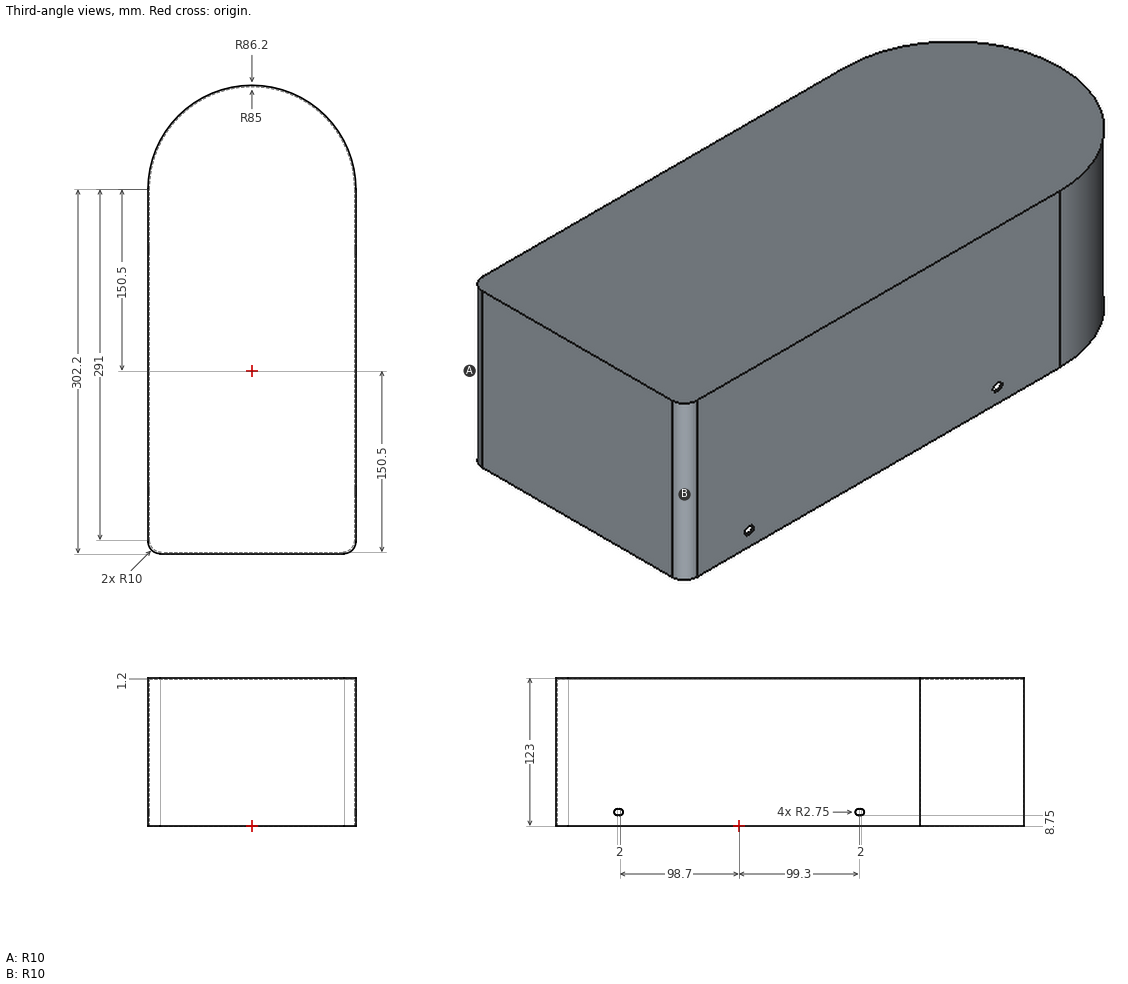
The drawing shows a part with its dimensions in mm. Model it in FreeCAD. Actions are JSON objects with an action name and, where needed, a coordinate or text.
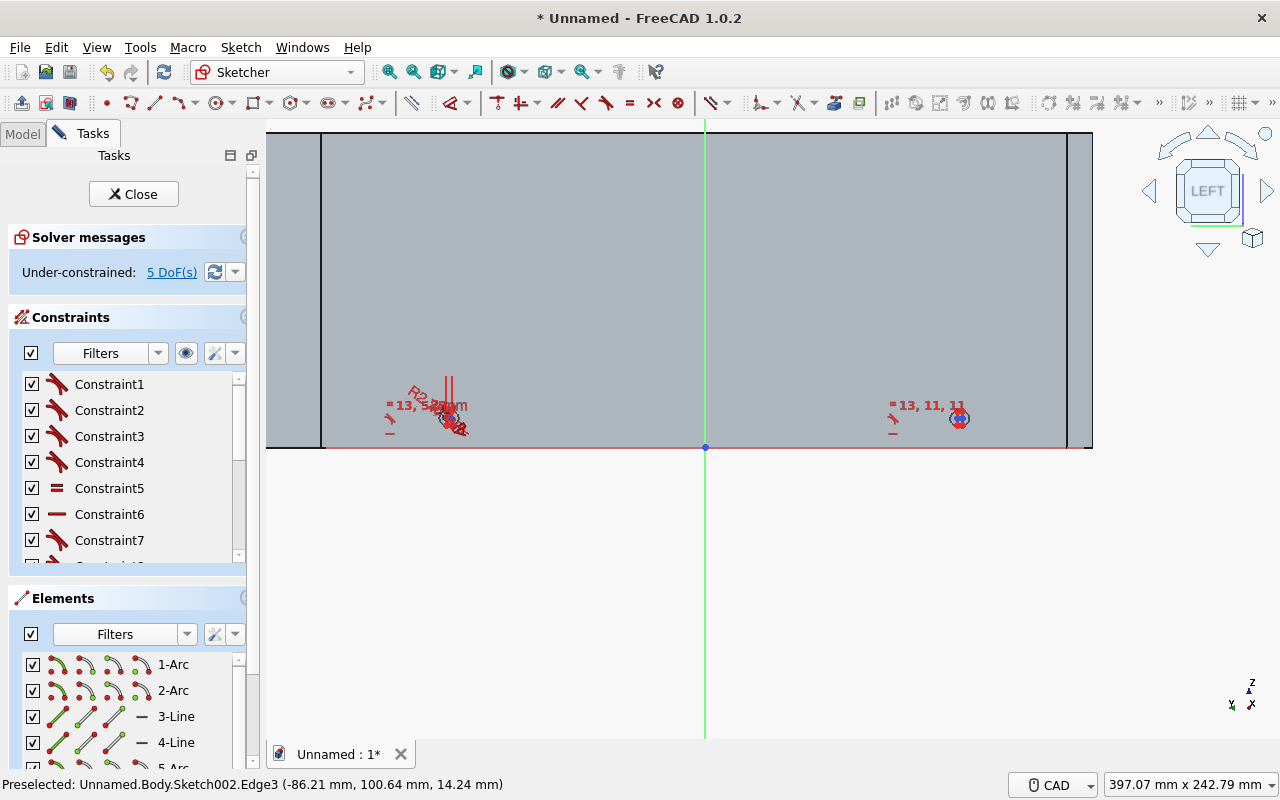
{"action": "scroll", "coordinate": [959, 412], "scroll_direction": "up", "scroll_amount": 11}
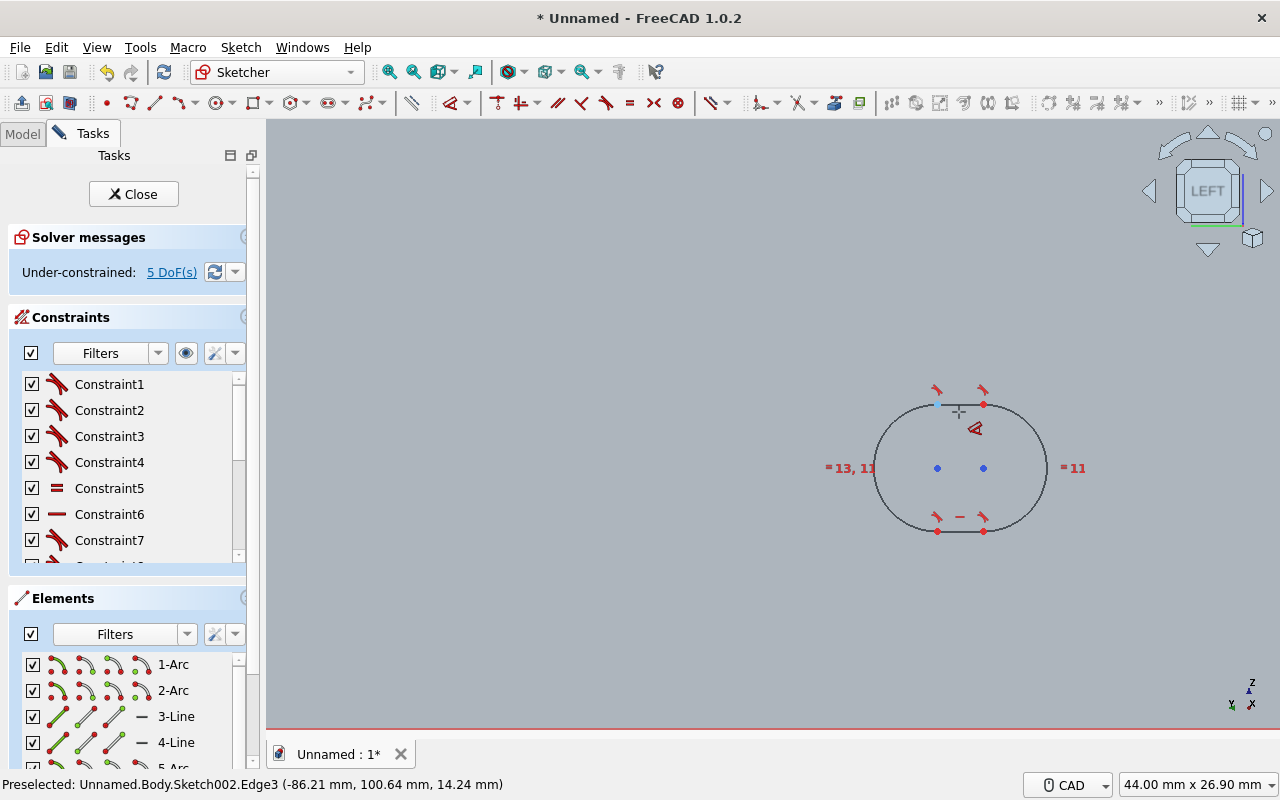
{"action": "left_click", "coordinate": [951, 405]}
{"action": "left_click", "coordinate": [960, 371]}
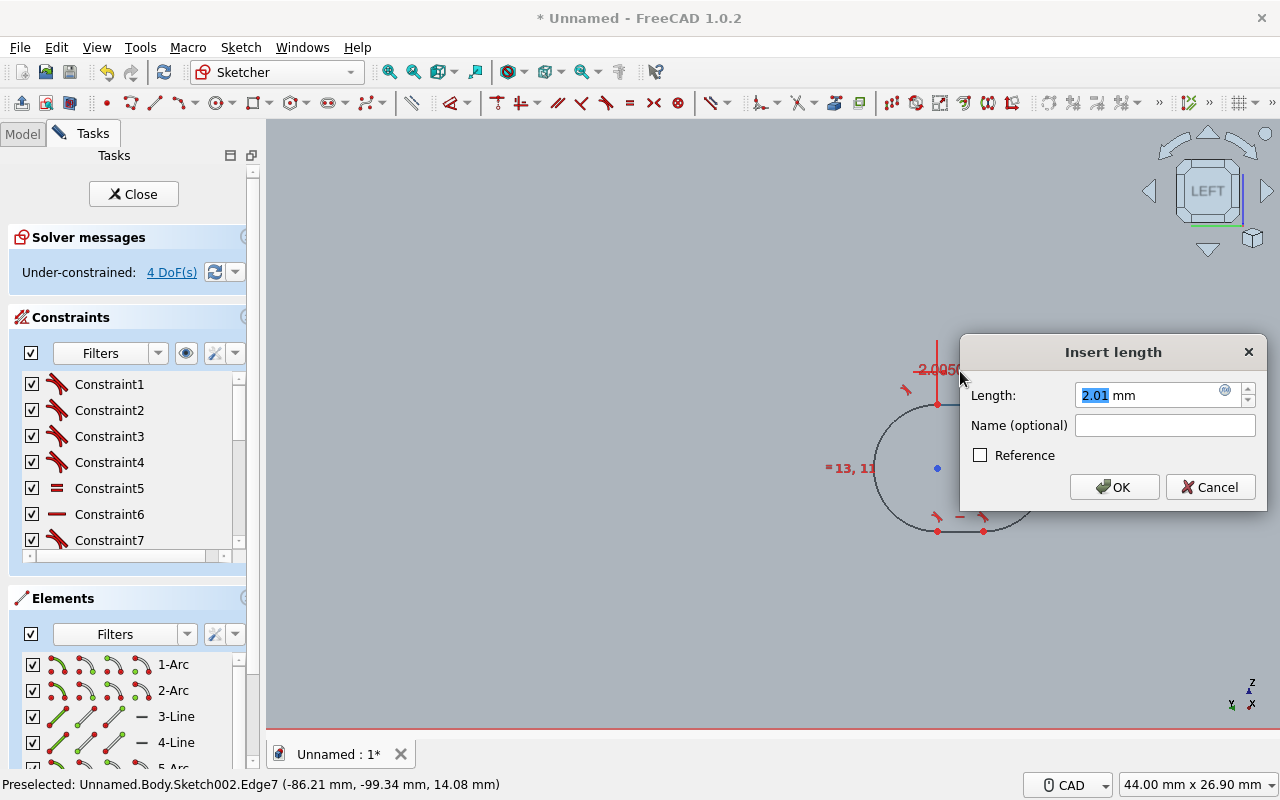
{"action": "type", "text": "2"}
{"action": "key", "text": "Return"}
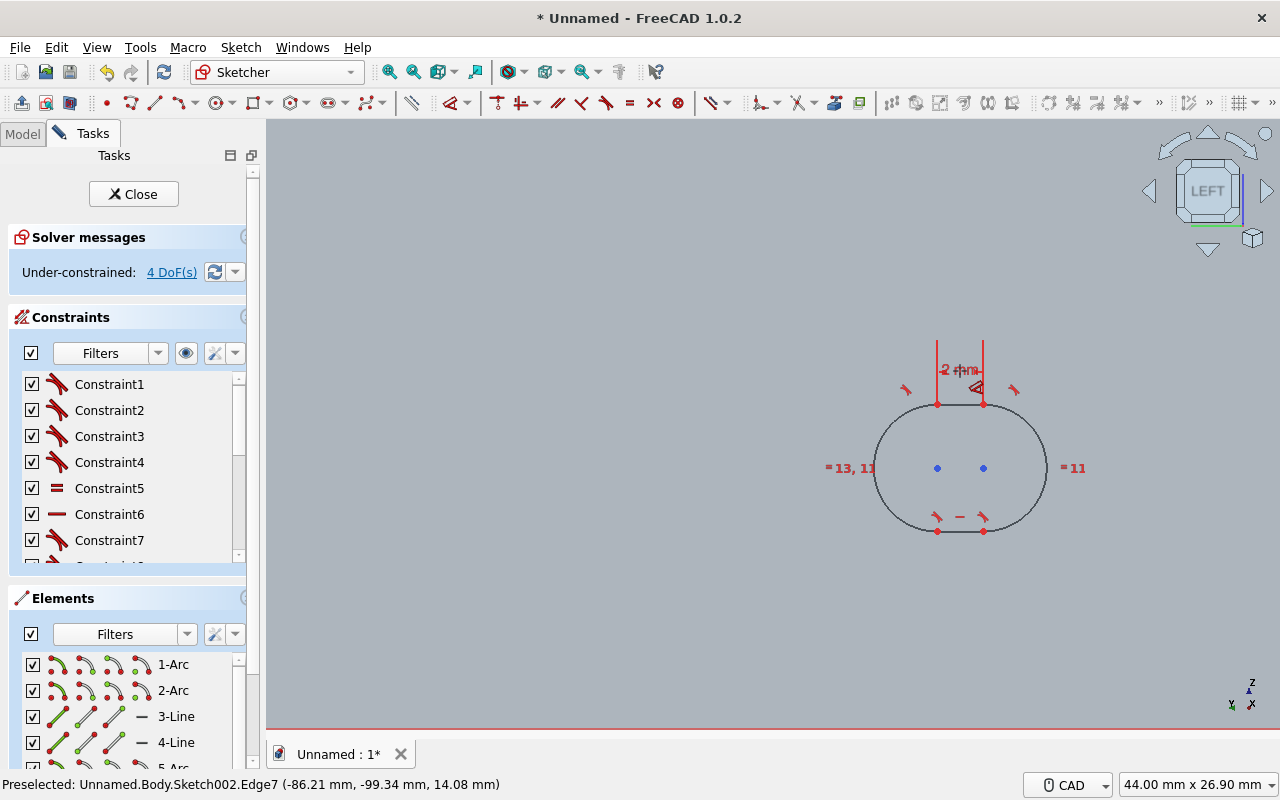
{"action": "scroll", "coordinate": [960, 412], "scroll_direction": "down", "scroll_amount": 11}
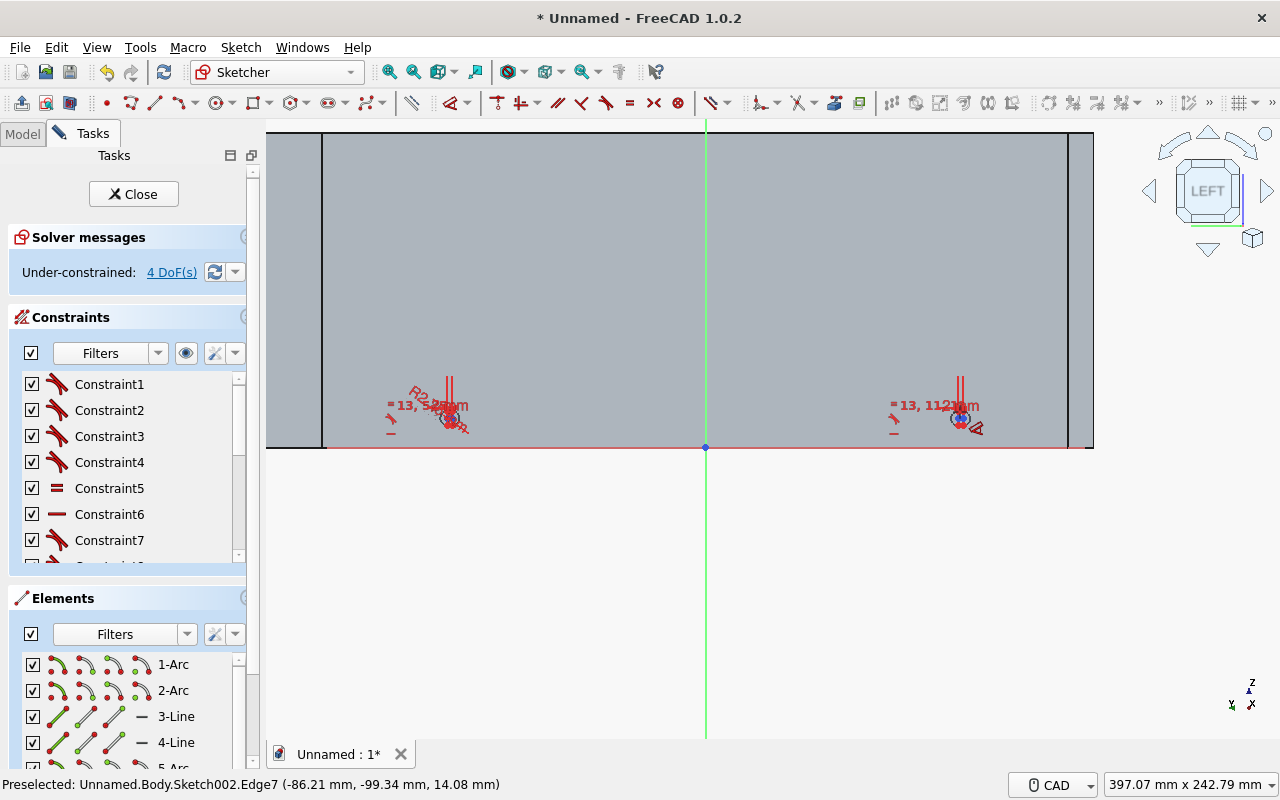
{"action": "scroll", "coordinate": [447, 425], "scroll_direction": "up", "scroll_amount": 5}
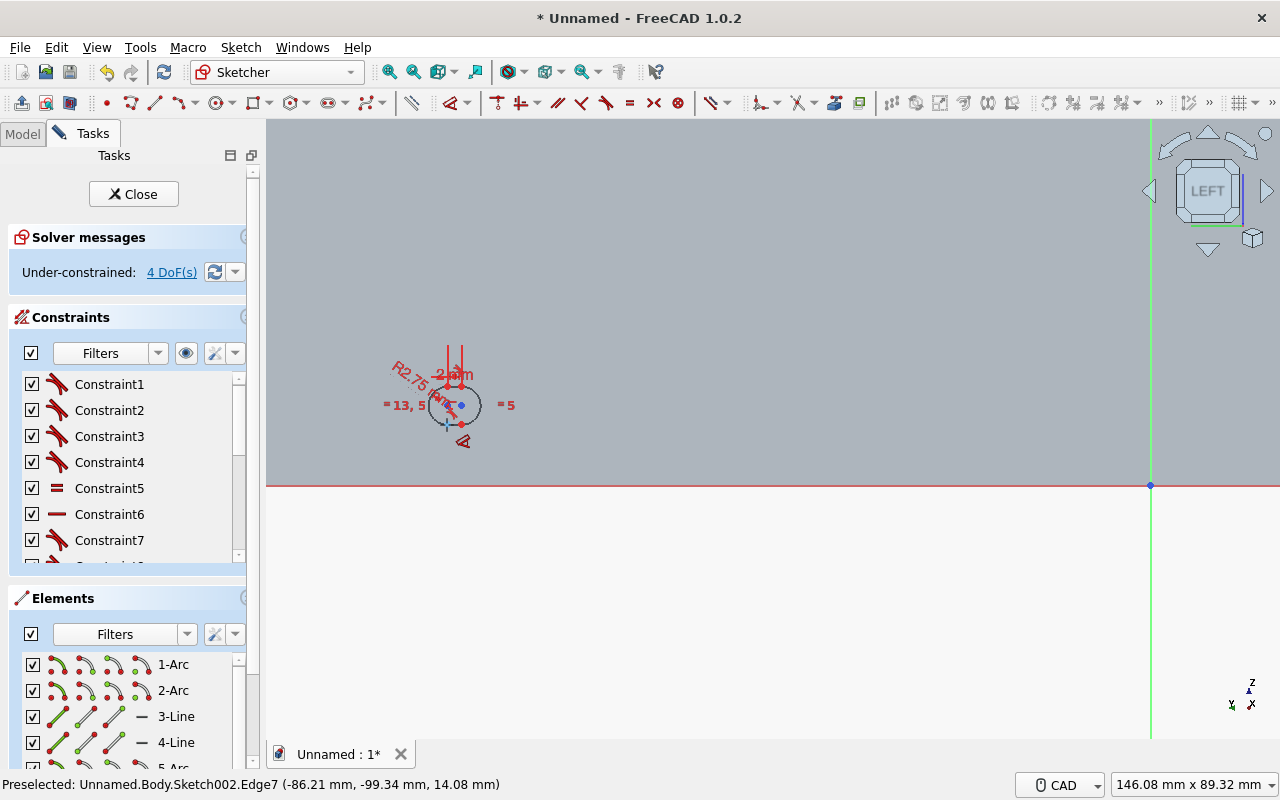
{"action": "left_click", "coordinate": [448, 425]}
{"action": "left_click", "coordinate": [414, 455]}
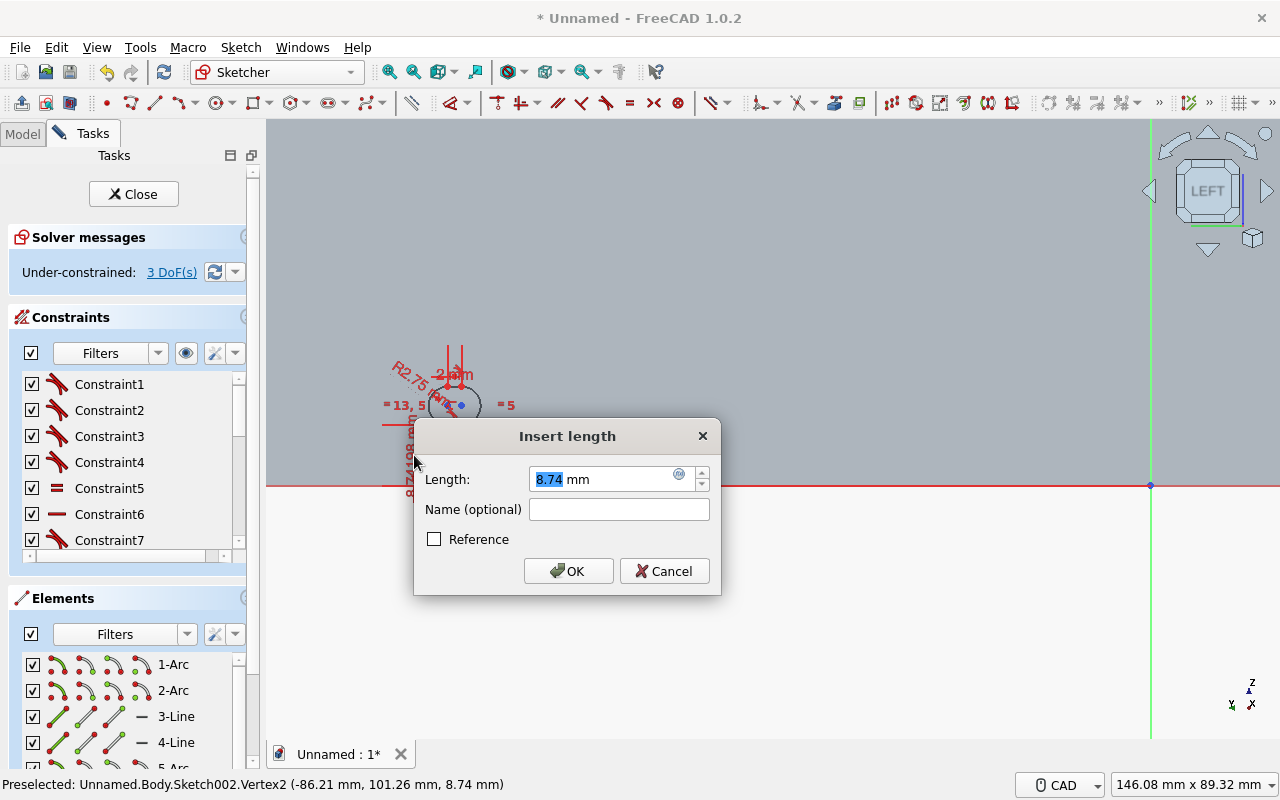
{"action": "type", "text": "8.75"}
{"action": "key", "text": "Return"}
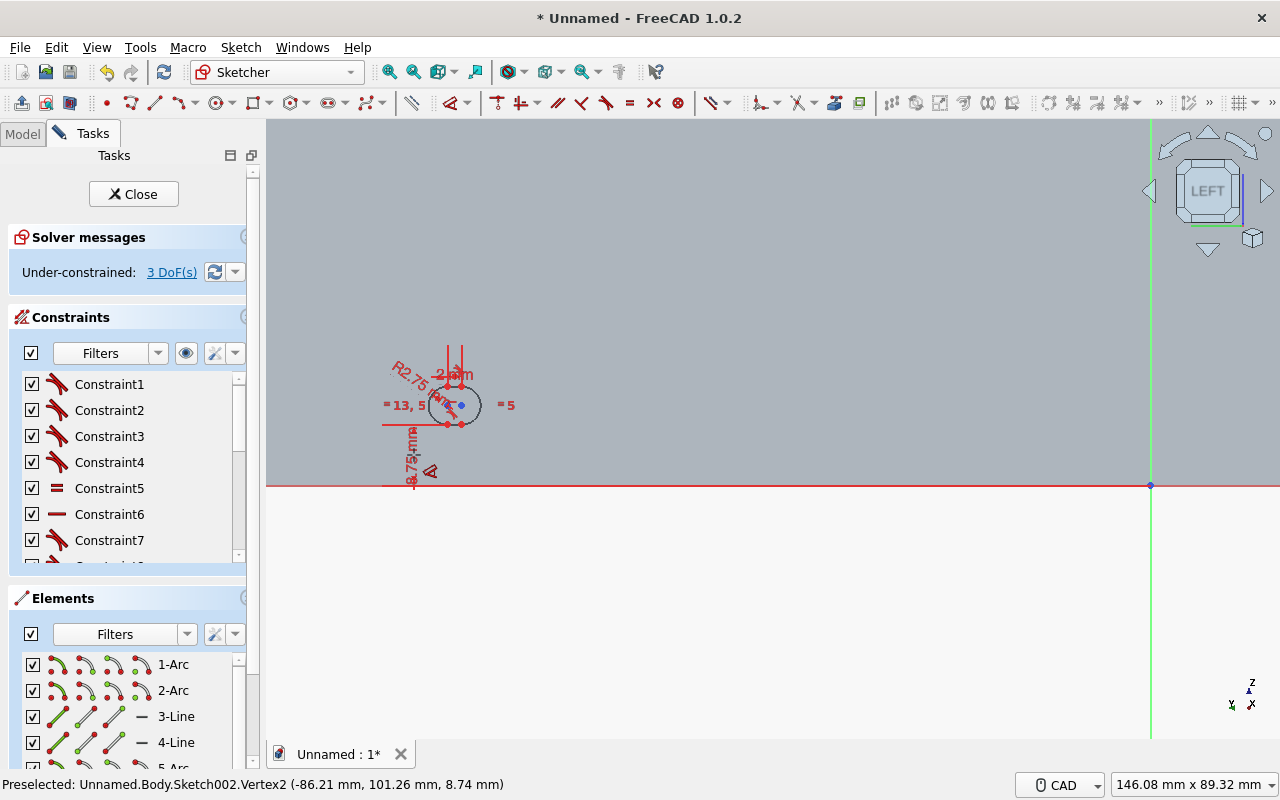
{"action": "left_click", "coordinate": [462, 425]}
{"action": "left_click", "coordinate": [788, 520]}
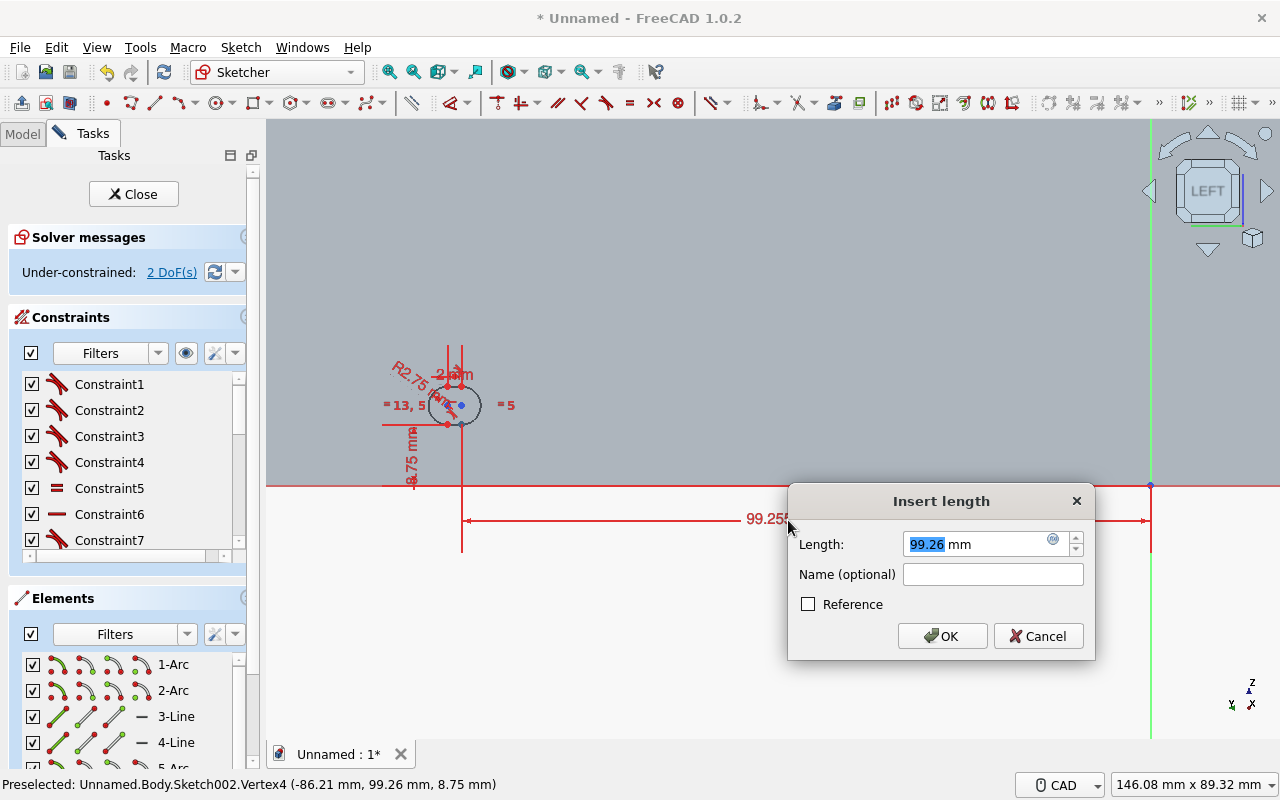
{"action": "type", "text": "99.3"}
{"action": "key", "text": "Return"}